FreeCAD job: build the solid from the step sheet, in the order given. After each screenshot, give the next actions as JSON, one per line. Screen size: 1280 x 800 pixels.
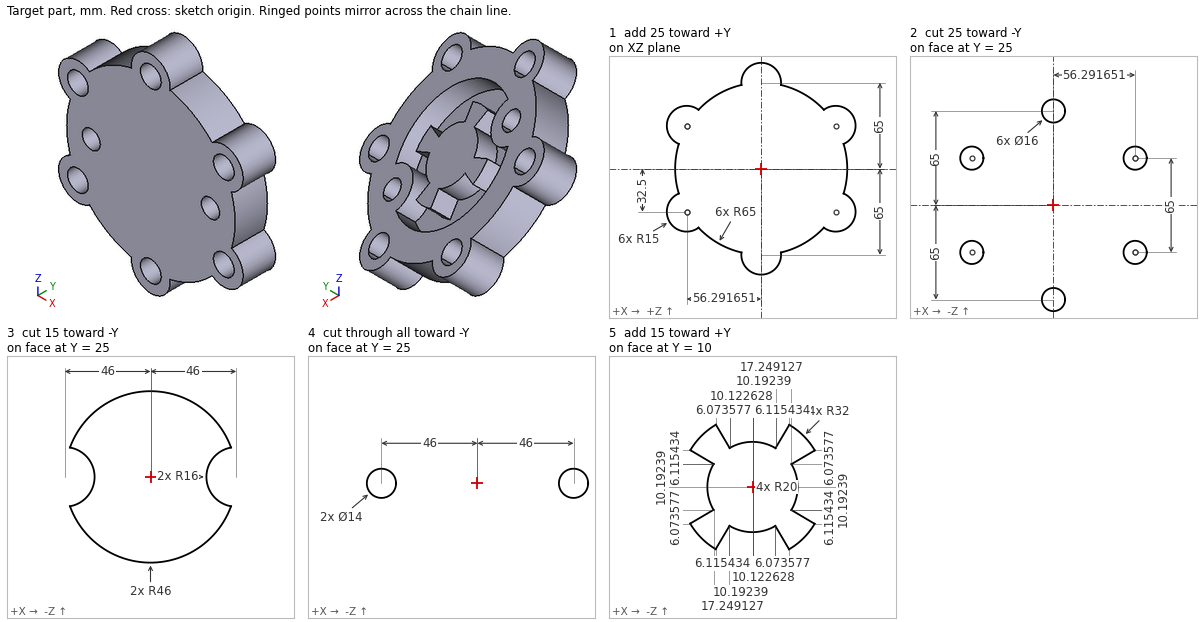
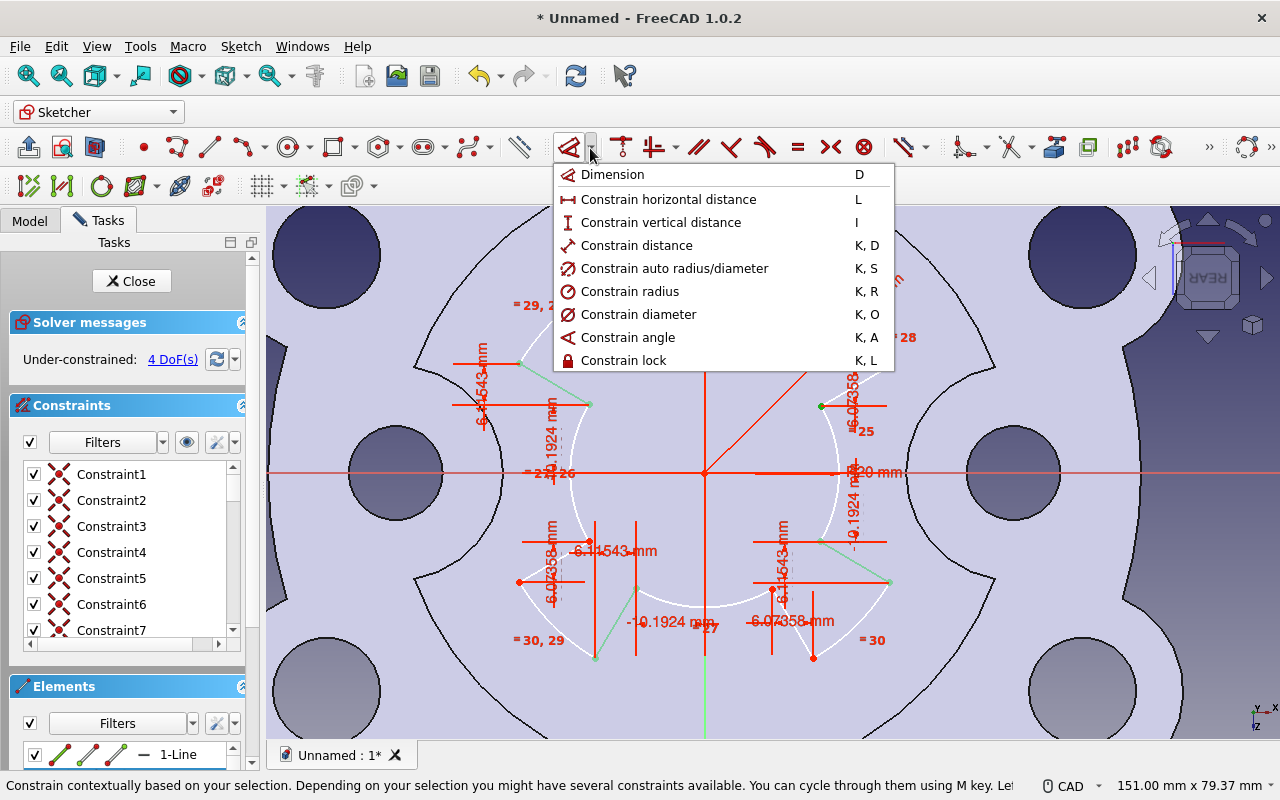
{"action": "left_click", "coordinate": [724, 200]}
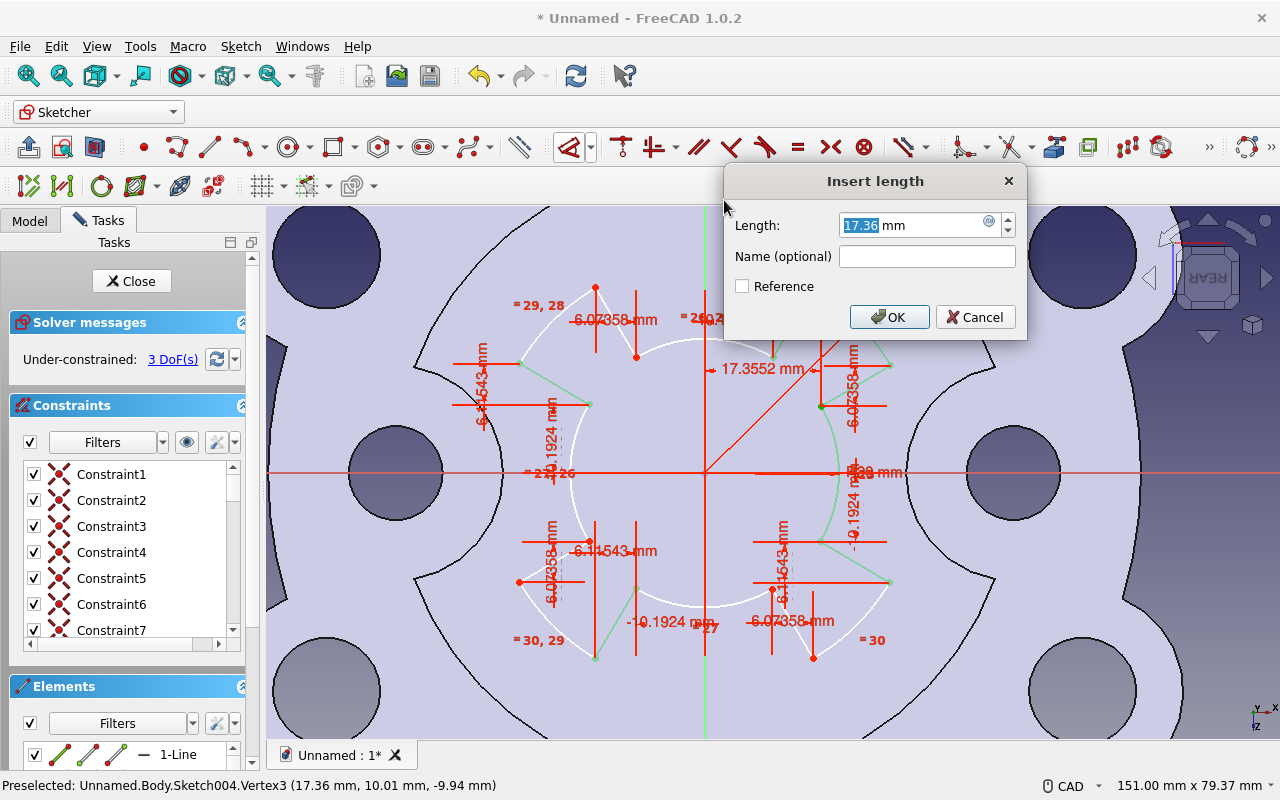
{"action": "type", "text": "17.249127"}
{"action": "key", "text": "Return"}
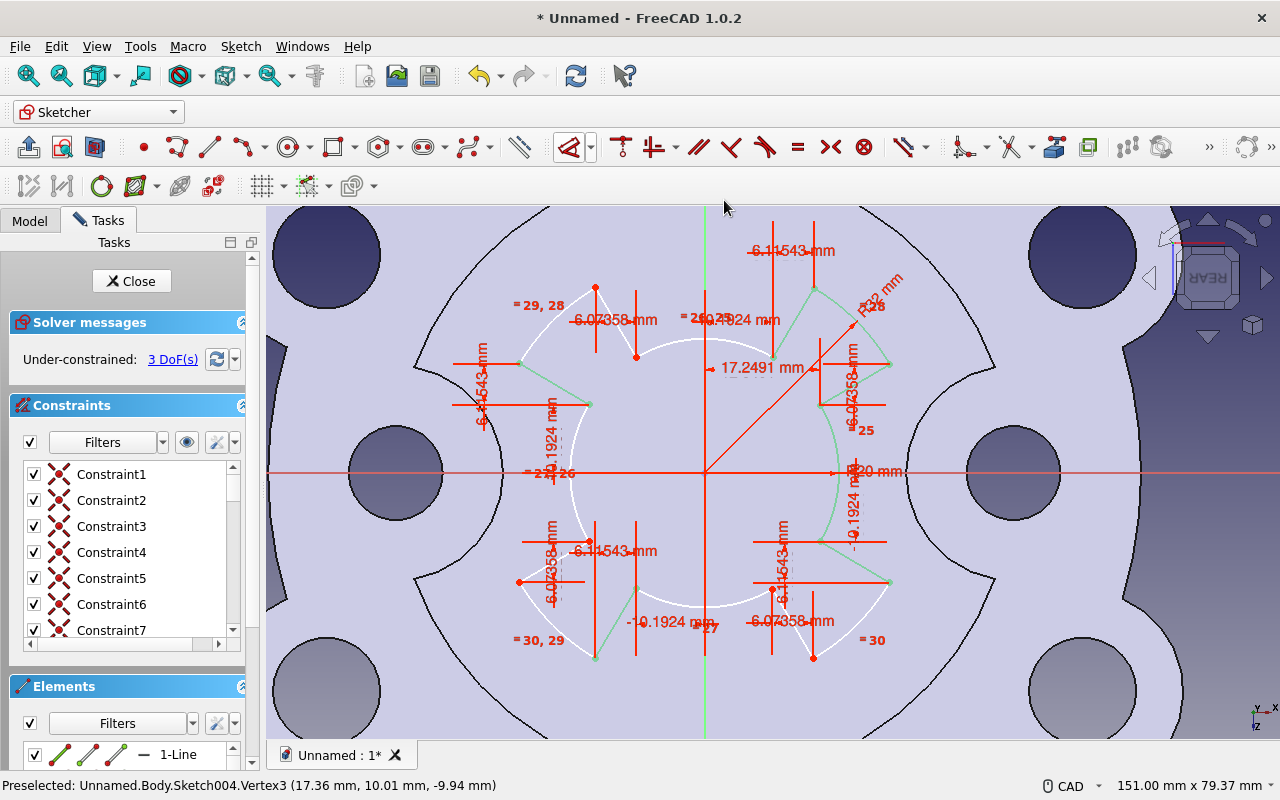
{"action": "left_click", "coordinate": [636, 357]}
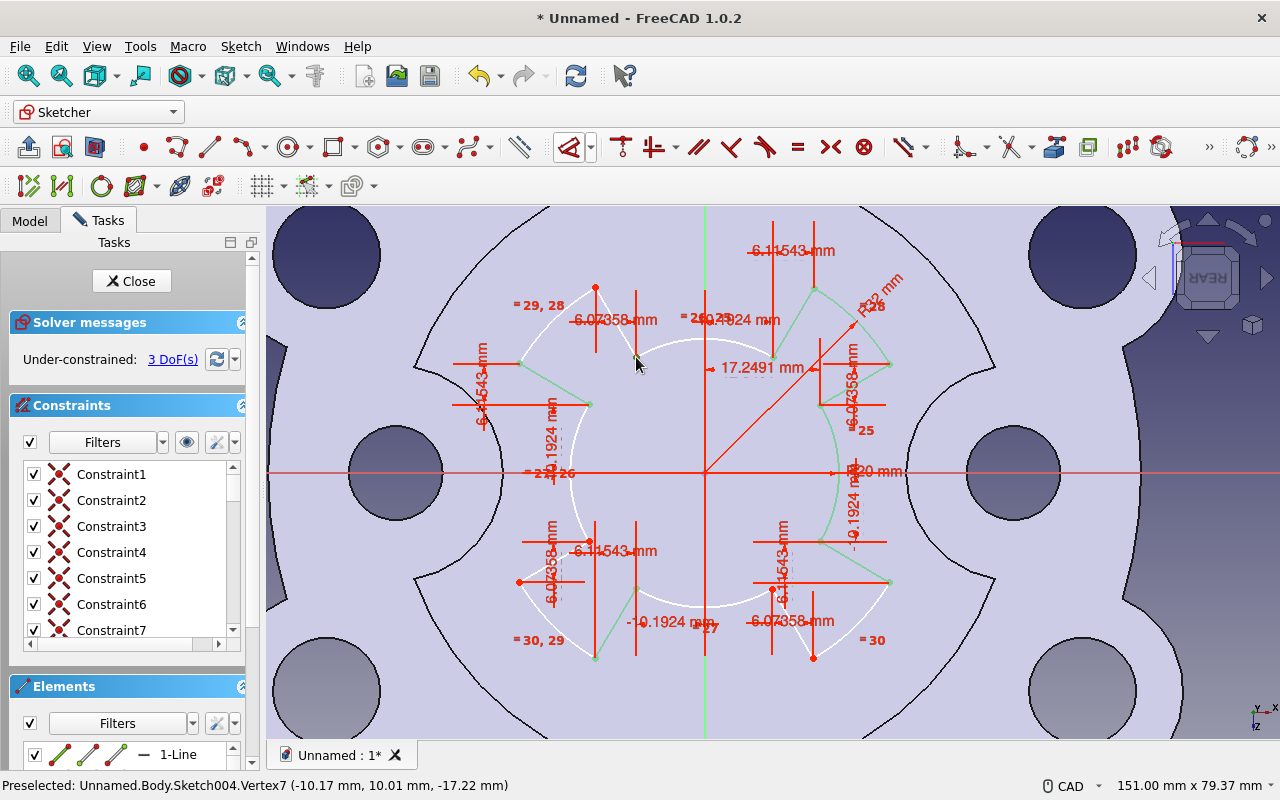
{"action": "left_click", "coordinate": [590, 148]}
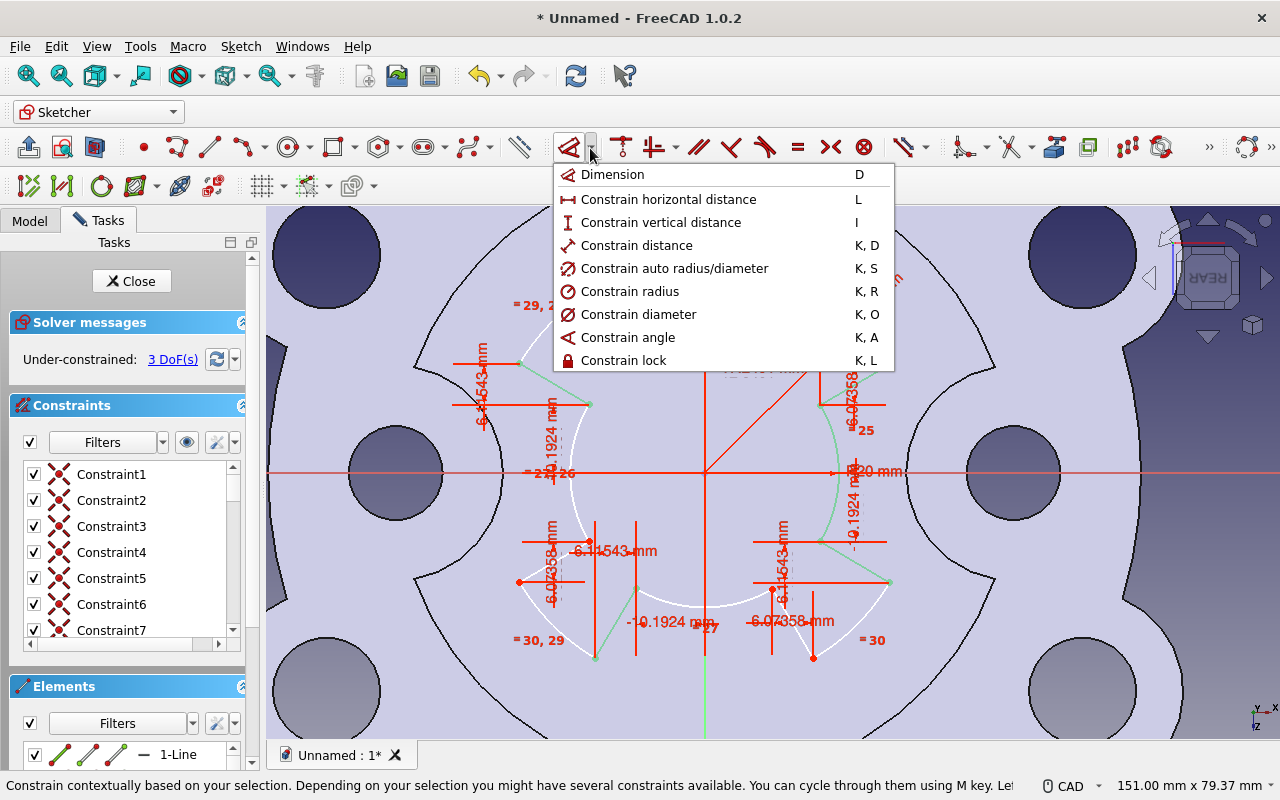
{"action": "left_click", "coordinate": [724, 200]}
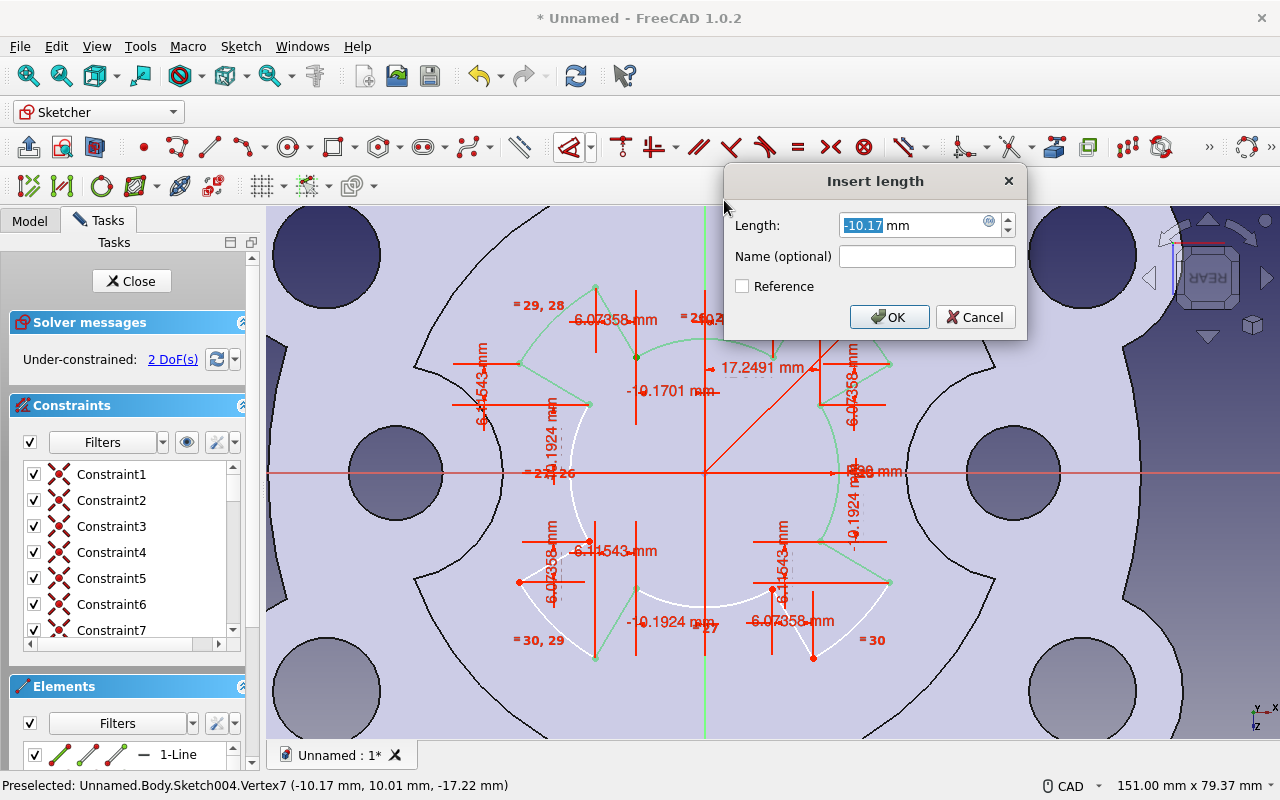
{"action": "type", "text": "-10.122628"}
{"action": "key", "text": "Return"}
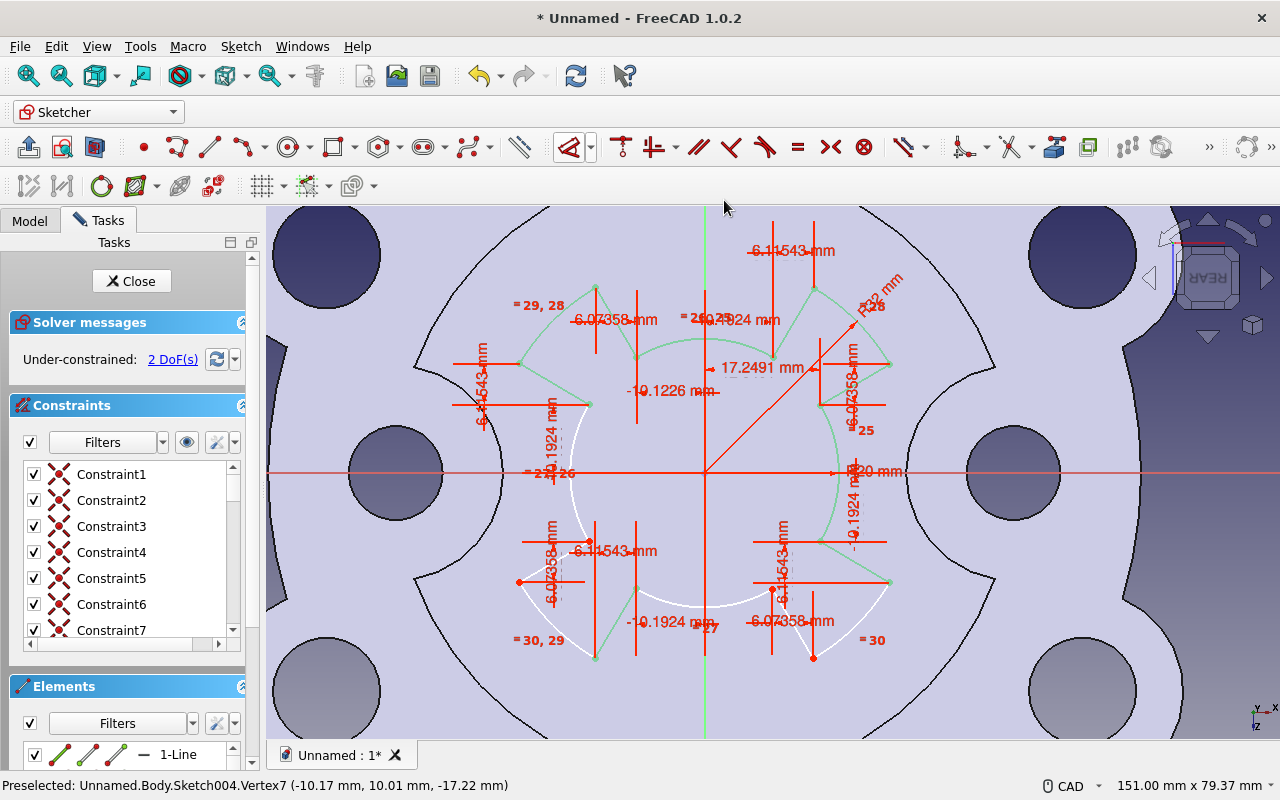
{"action": "left_click", "coordinate": [589, 542]}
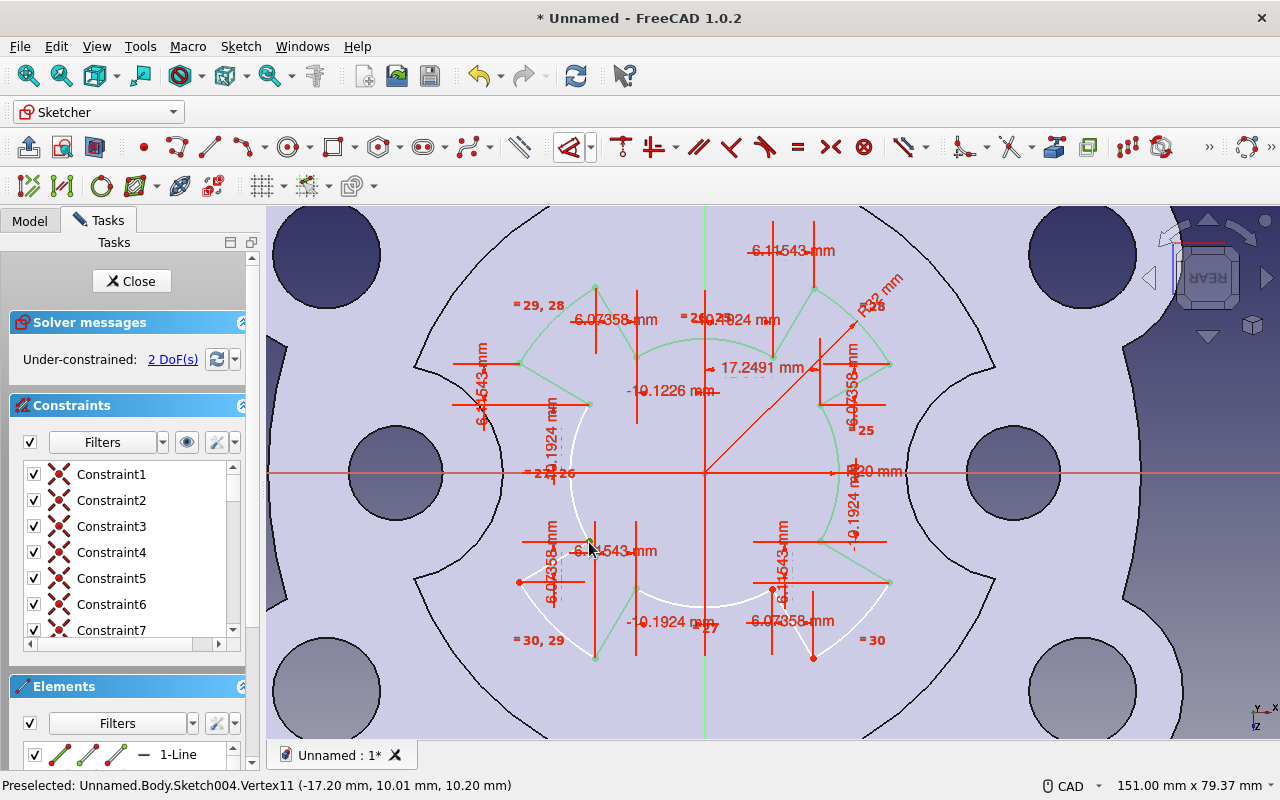
{"action": "left_click", "coordinate": [590, 148]}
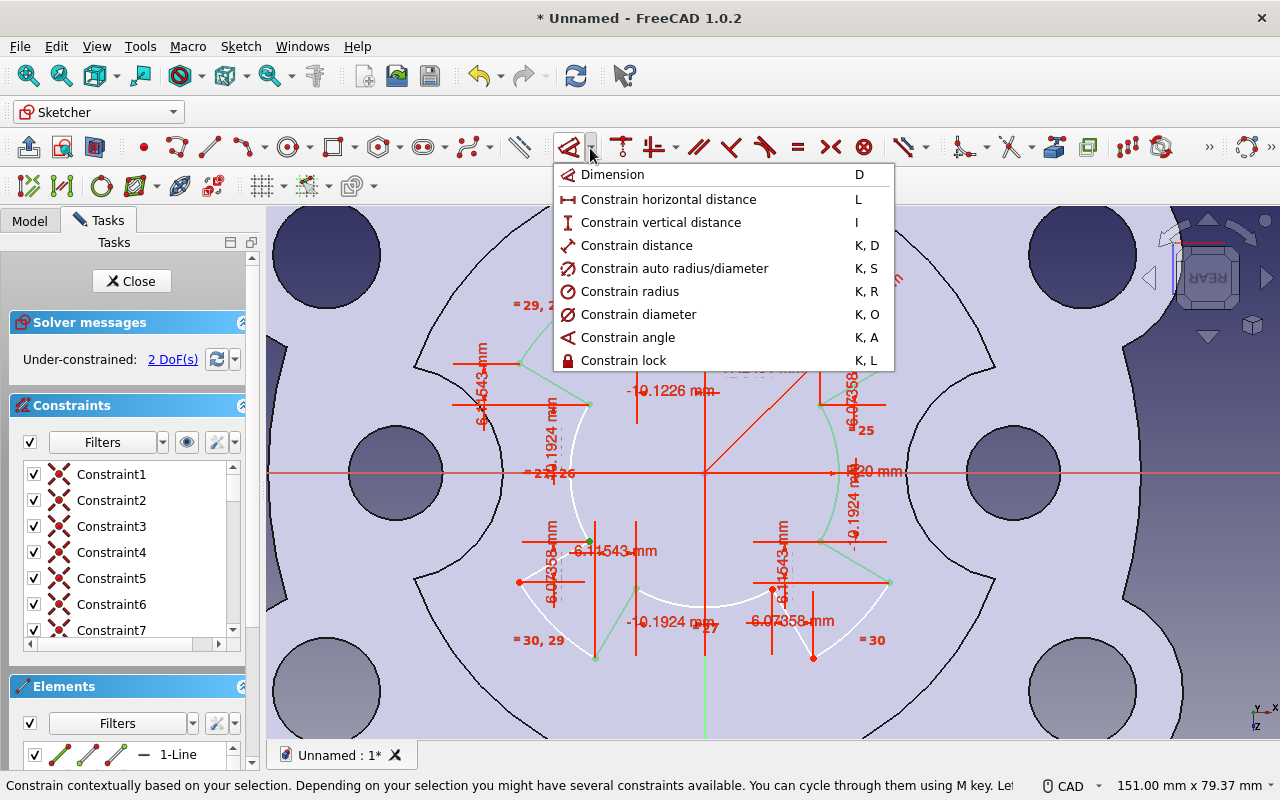
{"action": "left_click", "coordinate": [724, 200]}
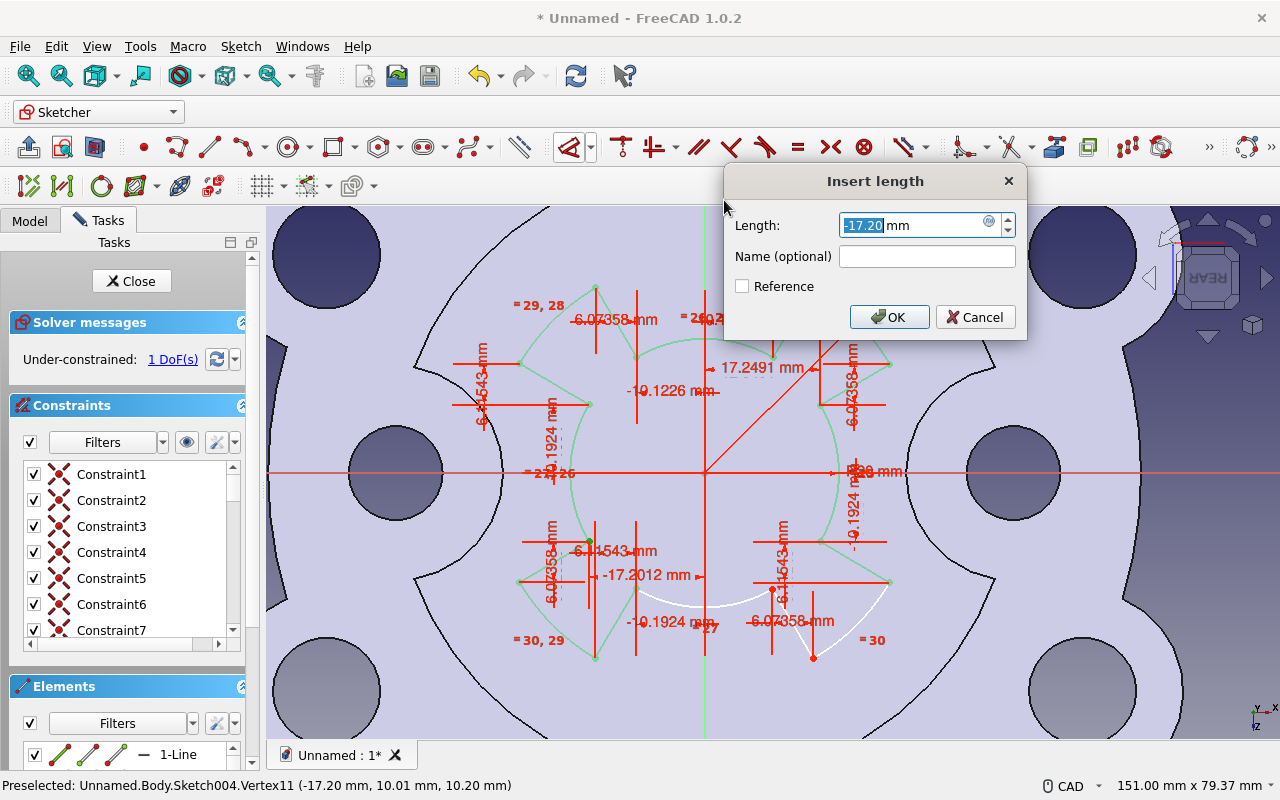
{"action": "type", "text": "-17.249127"}
{"action": "key", "text": "Return"}